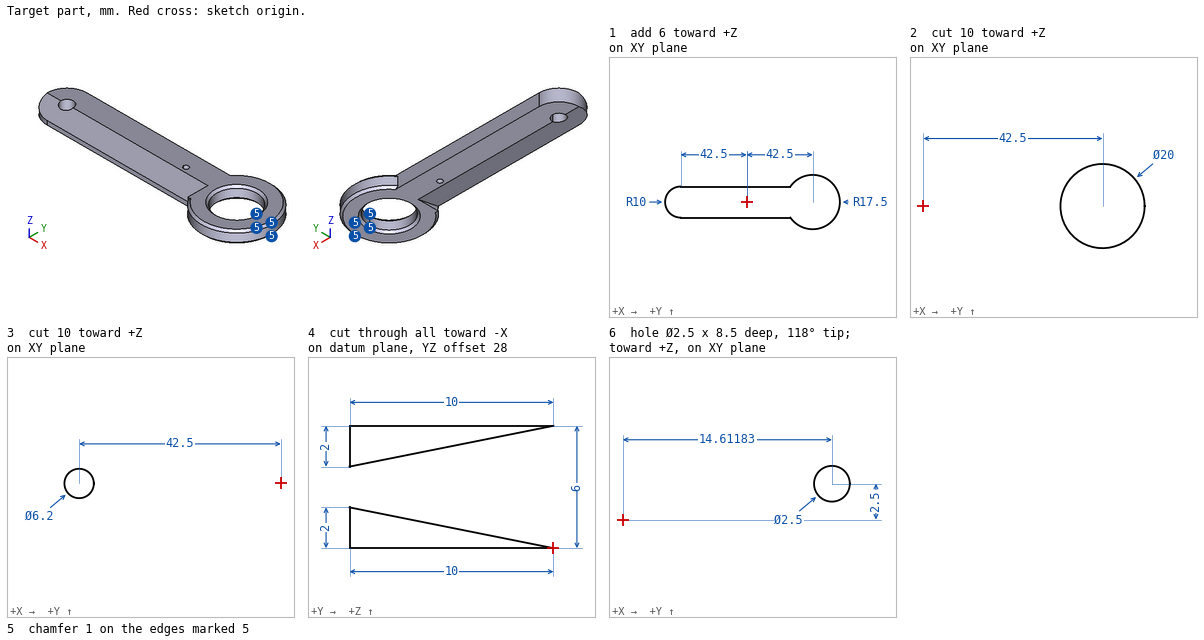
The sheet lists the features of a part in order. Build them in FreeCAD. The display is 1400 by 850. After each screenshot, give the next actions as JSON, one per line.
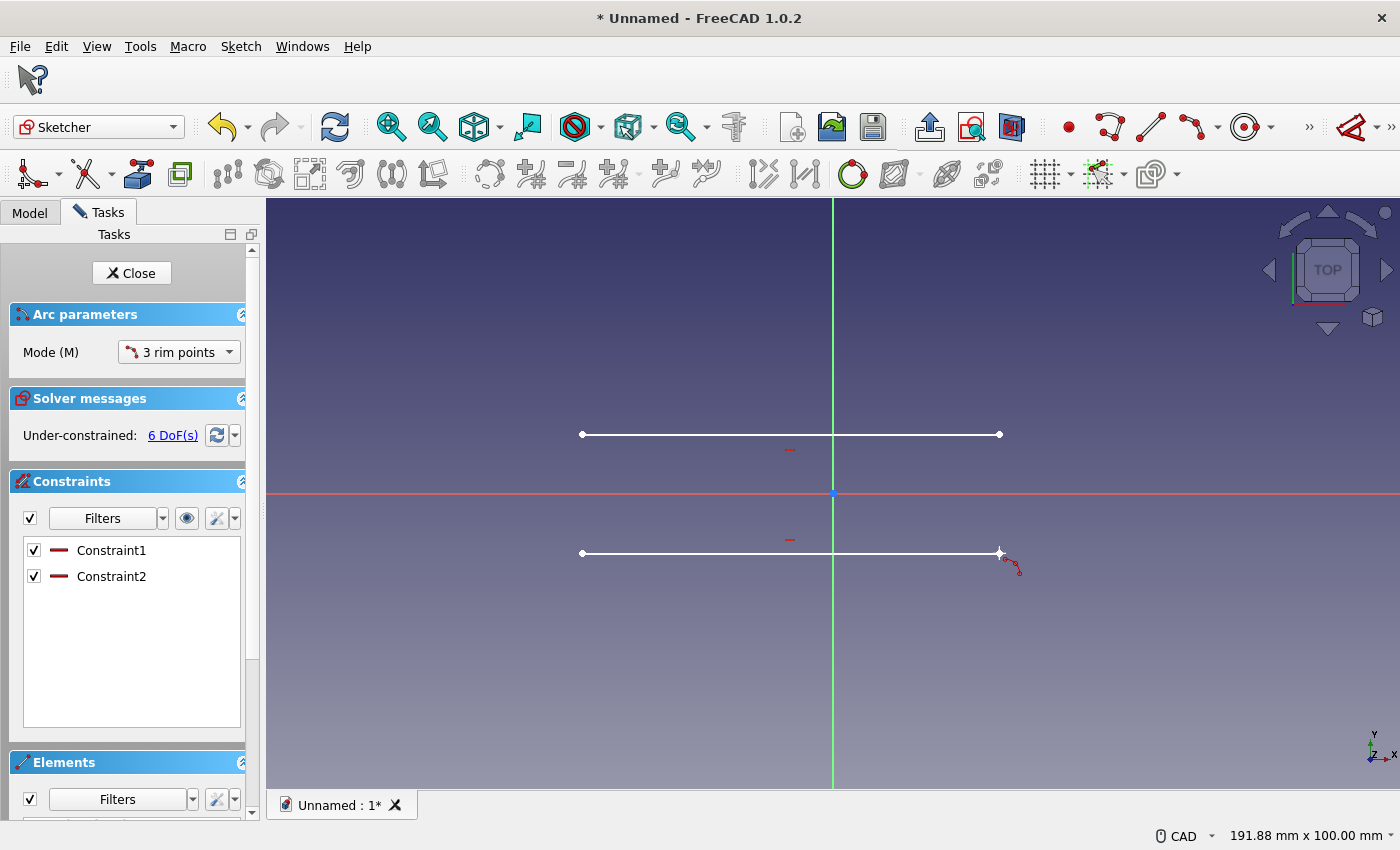
{"action": "left_click", "coordinate": [582, 435]}
{"action": "left_click", "coordinate": [582, 554]}
{"action": "left_click", "coordinate": [526, 475]}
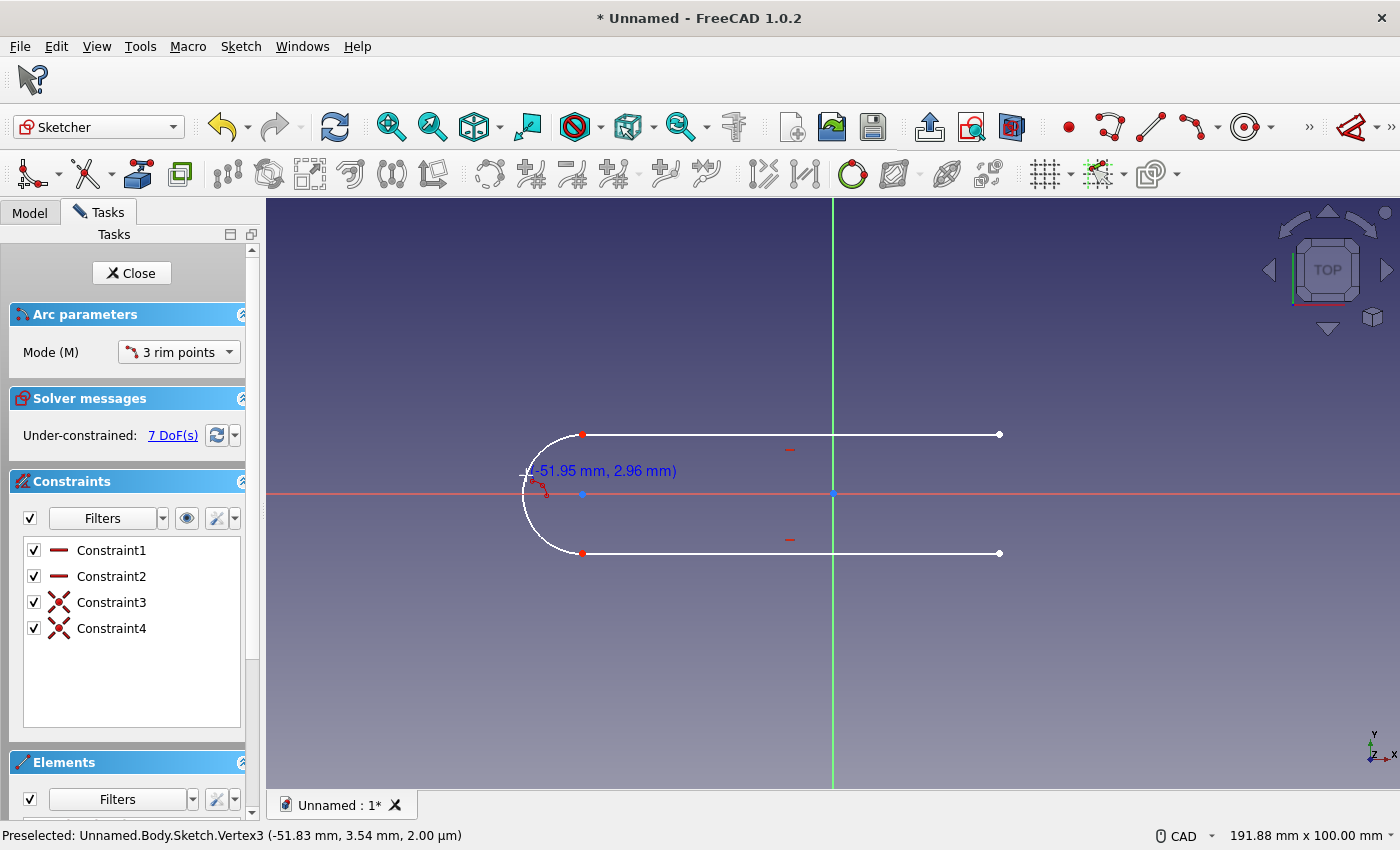
{"action": "left_click", "coordinate": [999, 554]}
{"action": "left_click", "coordinate": [999, 435]}
{"action": "left_click", "coordinate": [1175, 544]}
{"action": "key", "text": "Escape"}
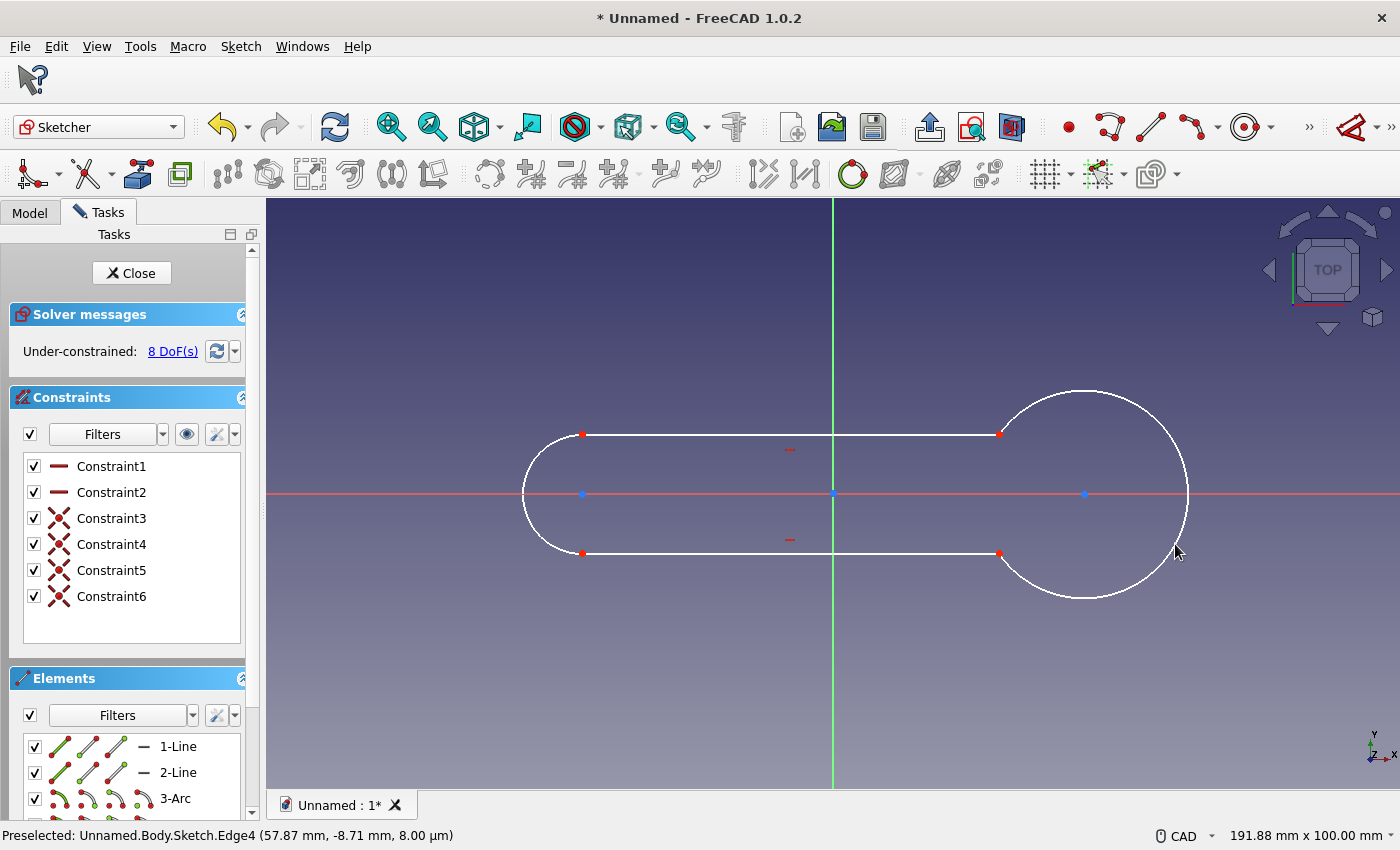
{"action": "left_click", "coordinate": [874, 435]}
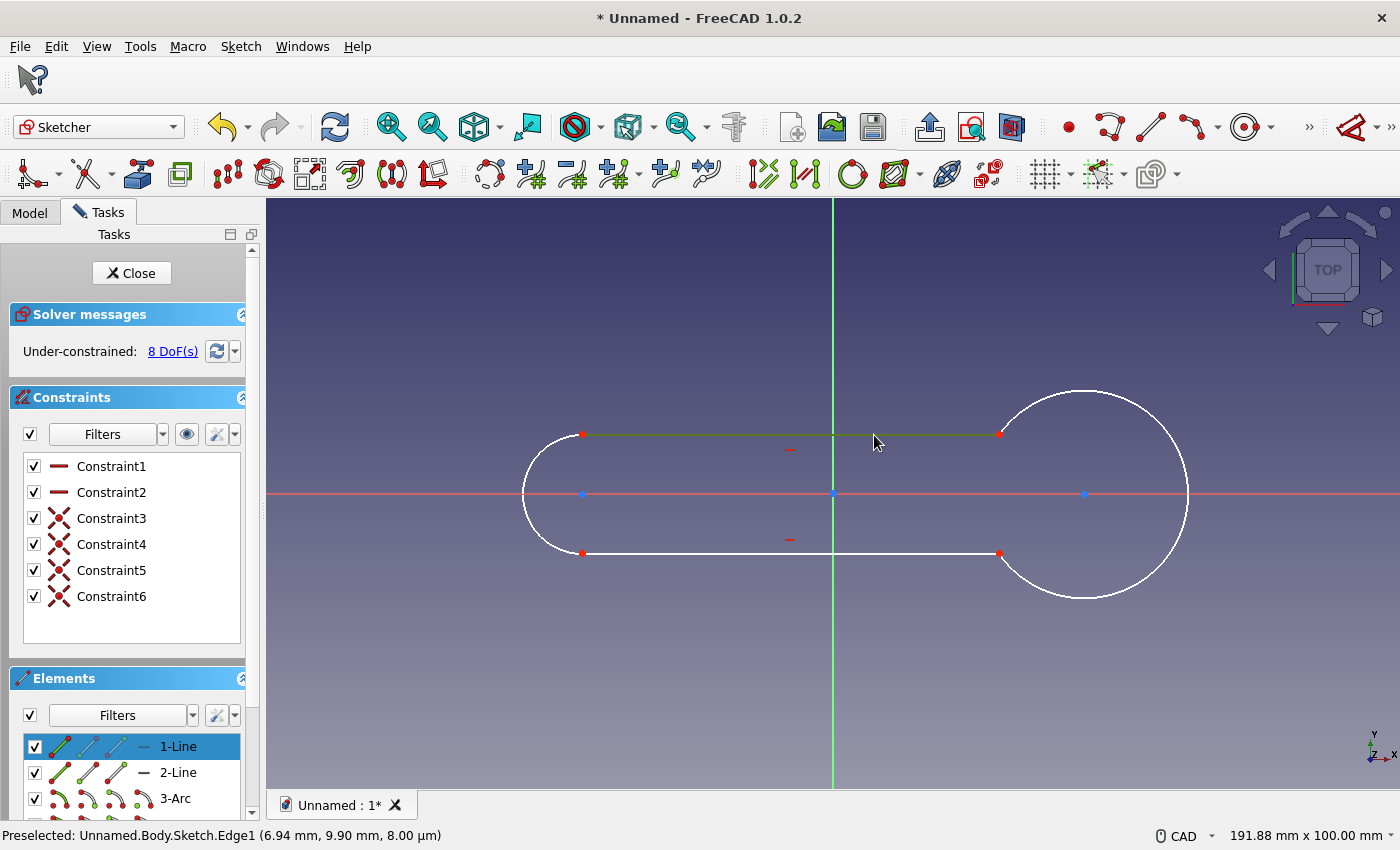
{"action": "left_click", "coordinate": [534, 460]}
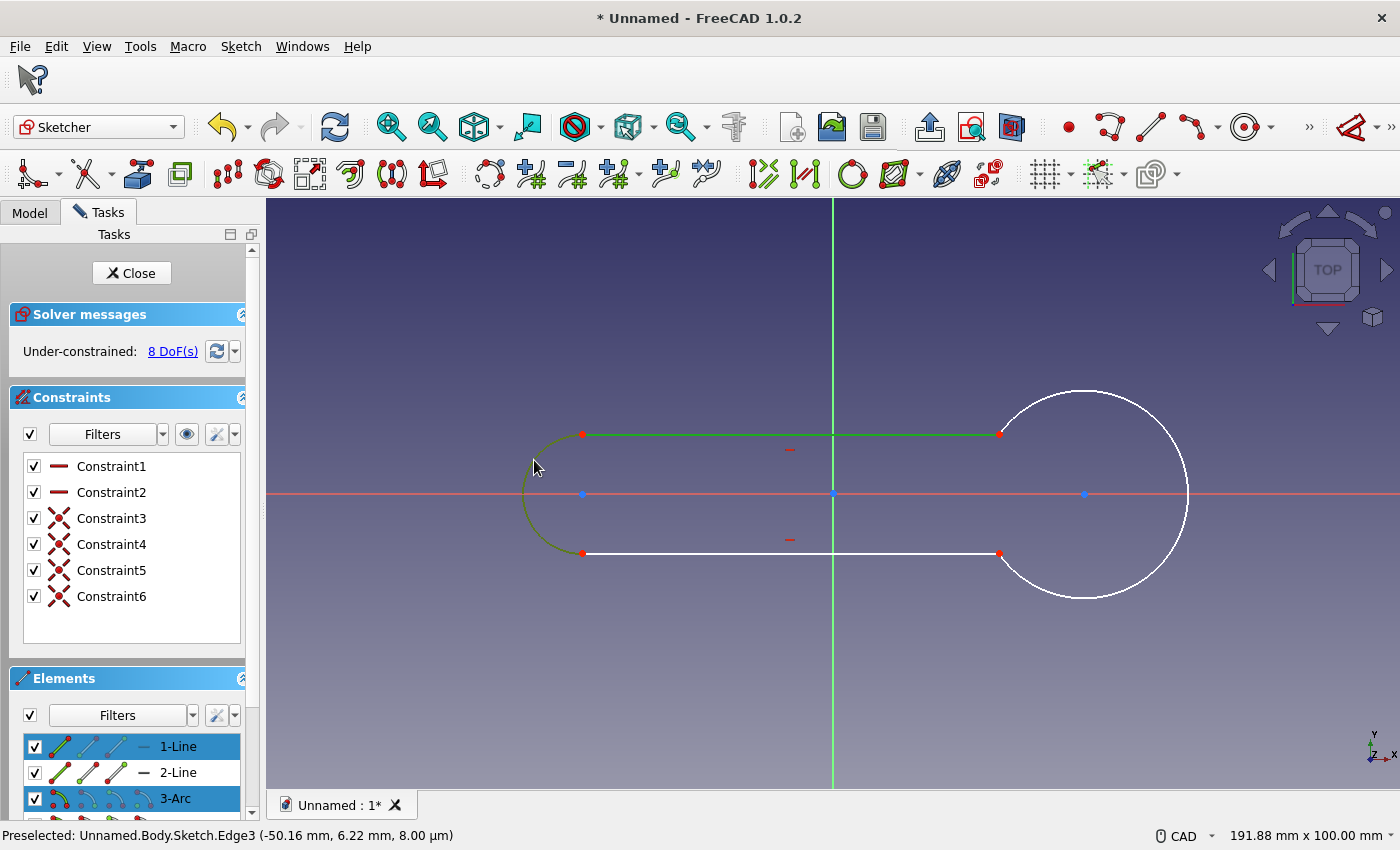
{"action": "key", "text": "t"}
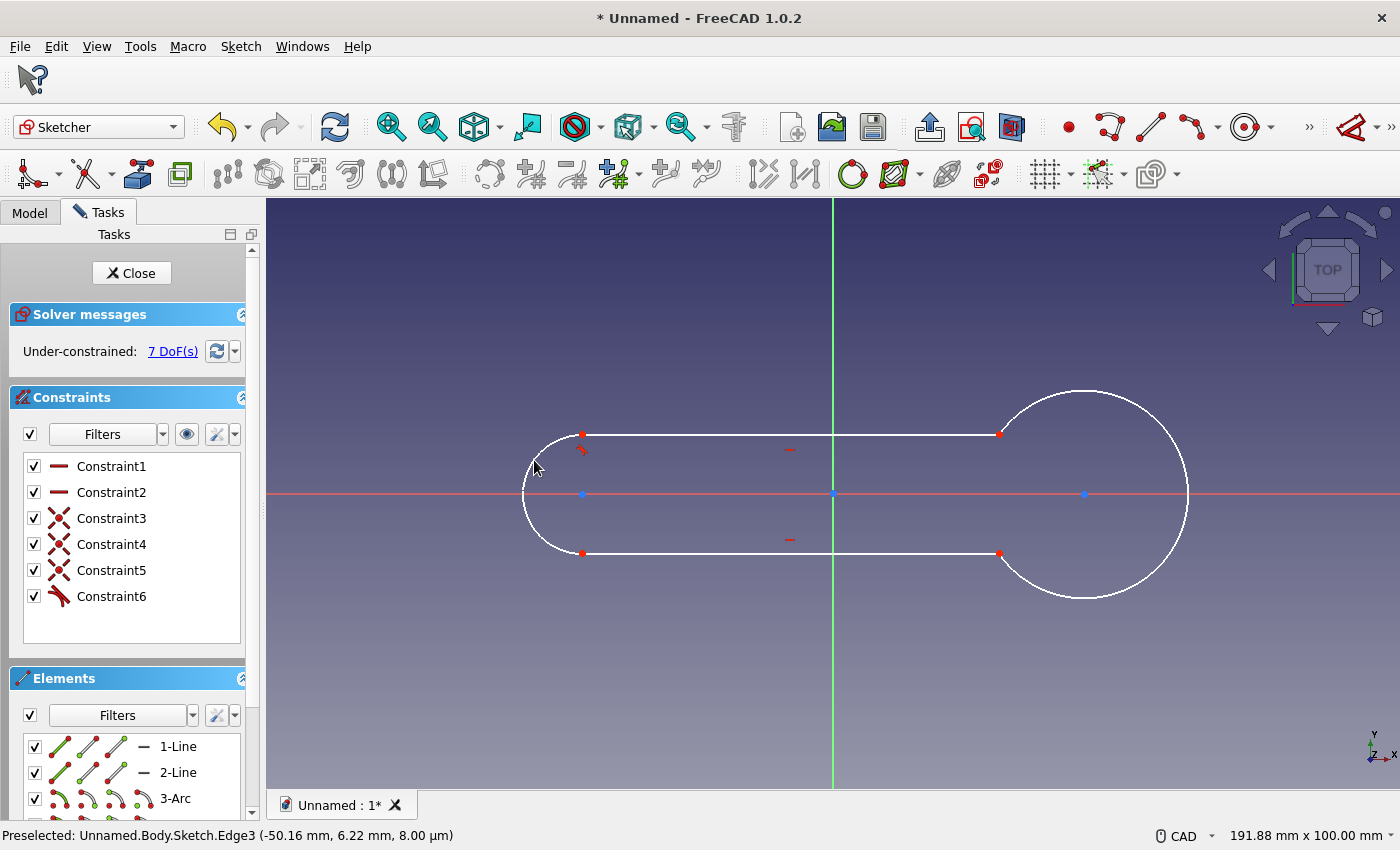
{"action": "left_click", "coordinate": [707, 554]}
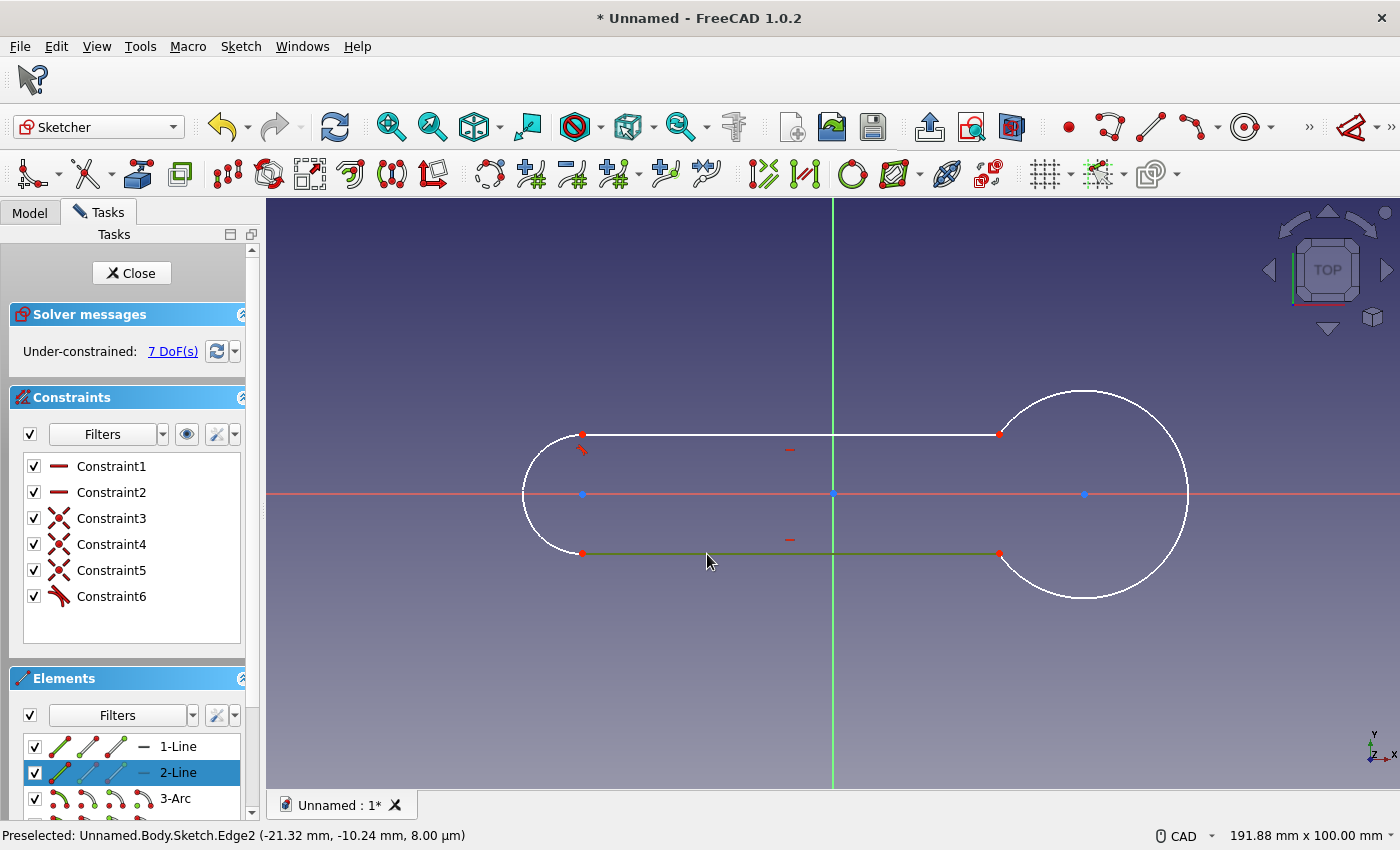
{"action": "left_click", "coordinate": [535, 459]}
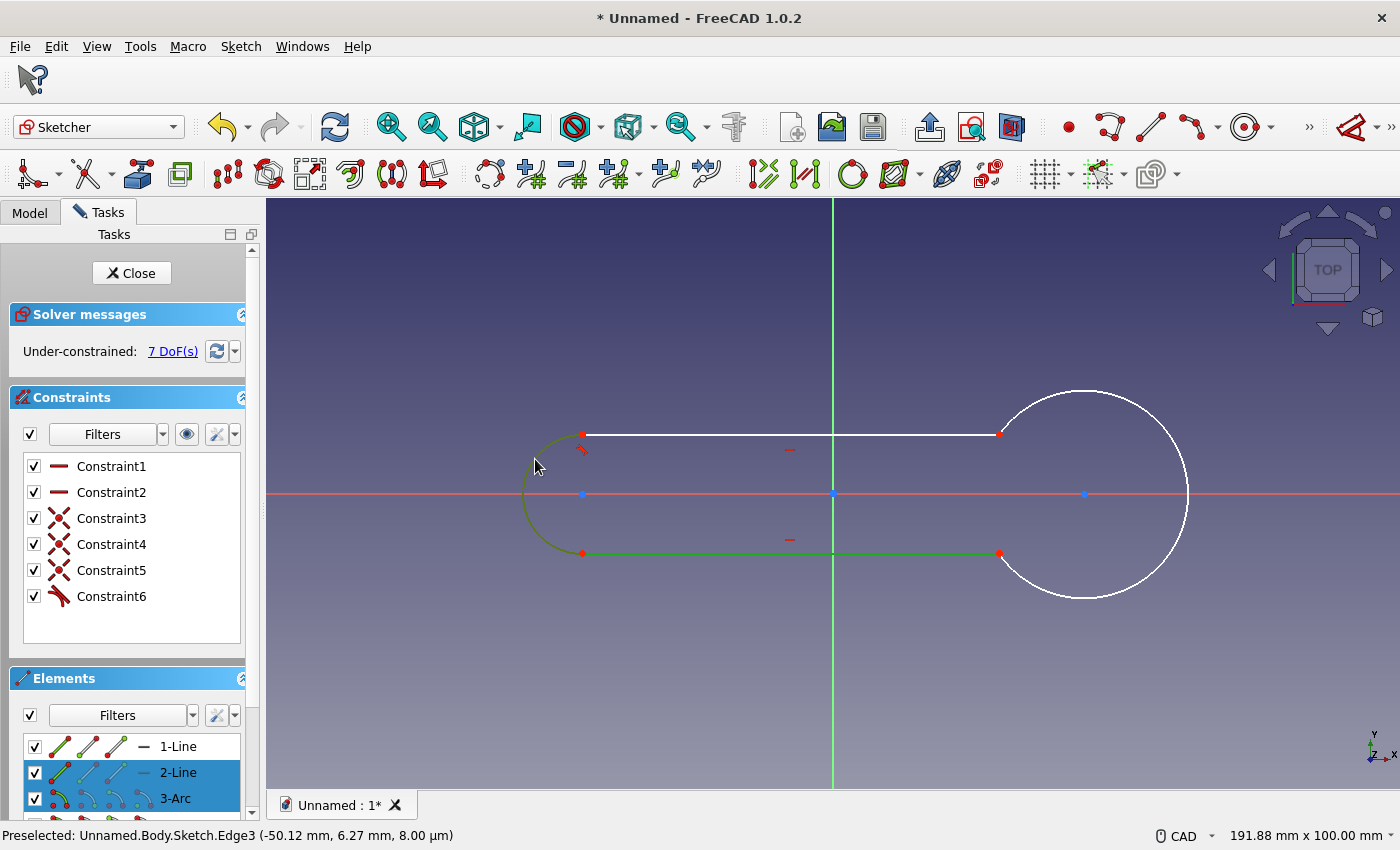
{"action": "key", "text": "t"}